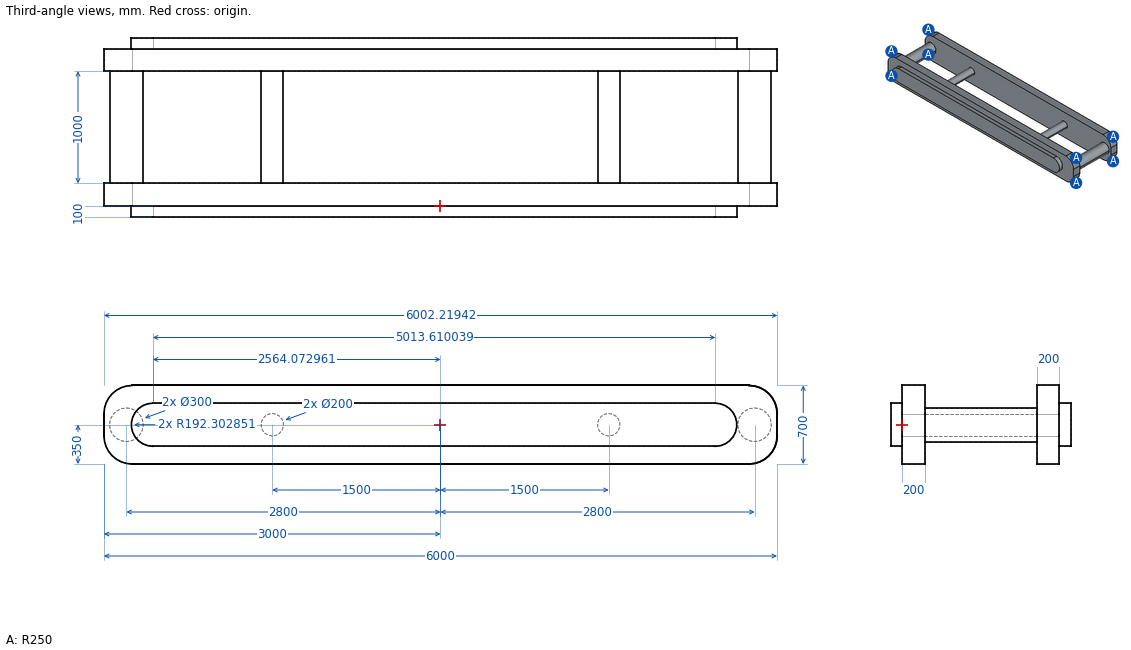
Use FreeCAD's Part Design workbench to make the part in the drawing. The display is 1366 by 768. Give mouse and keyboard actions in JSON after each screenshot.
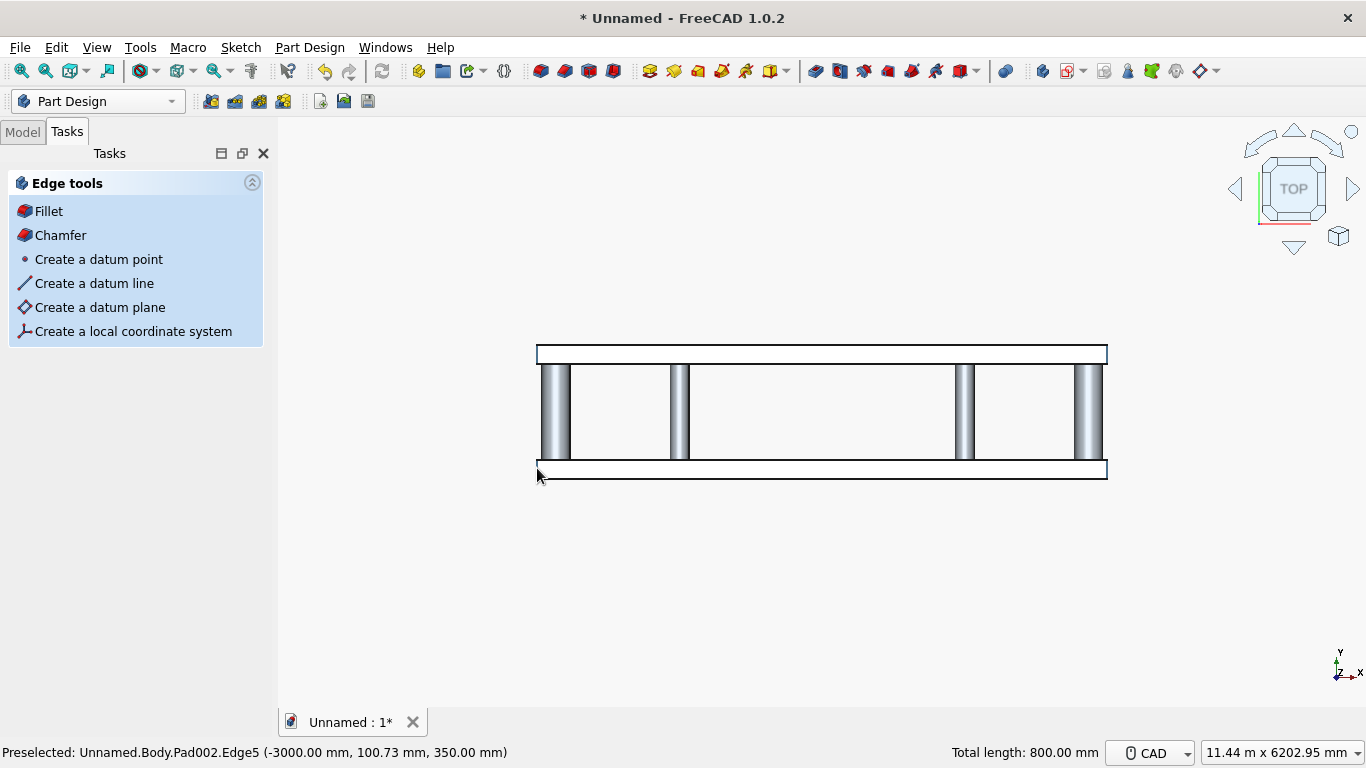
{"action": "scroll", "coordinate": [1107, 354], "scroll_direction": "up", "scroll_amount": 4}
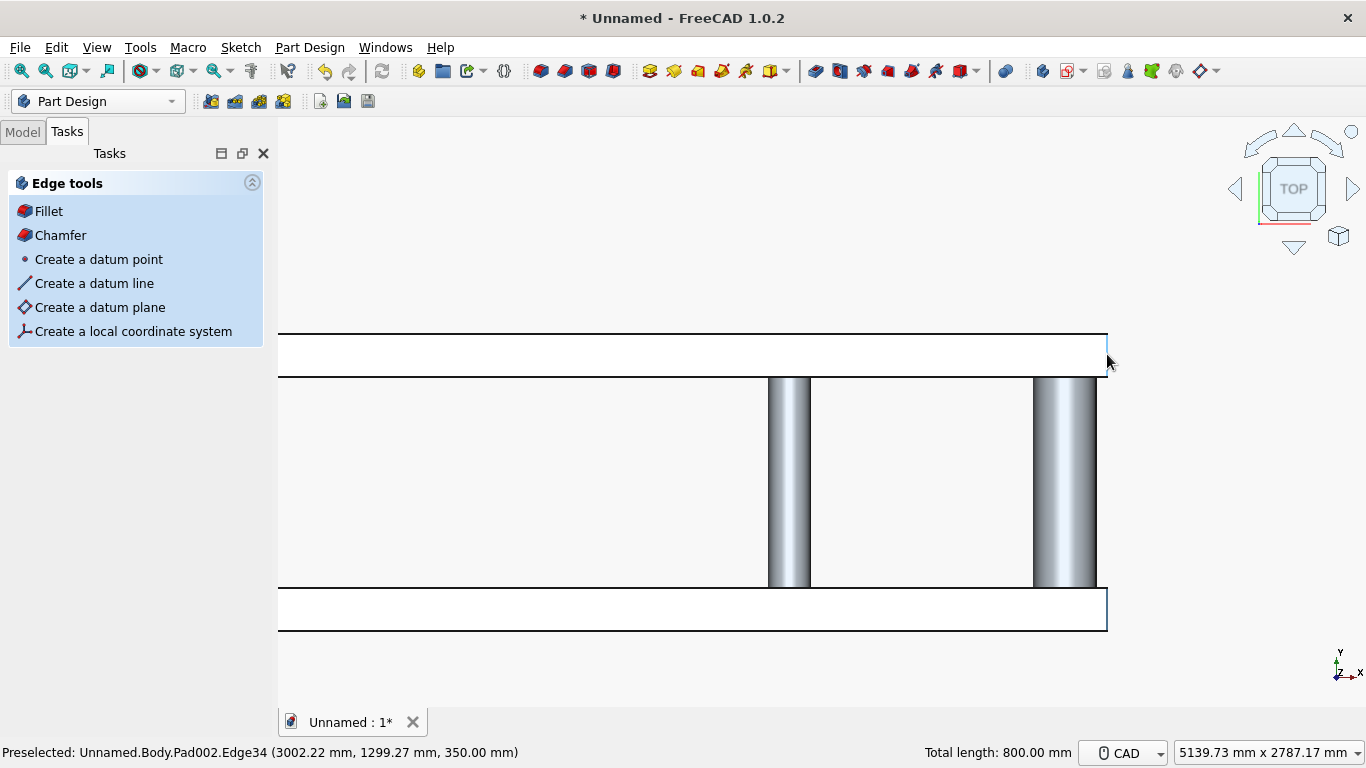
{"action": "left_click", "coordinate": [22, 72]}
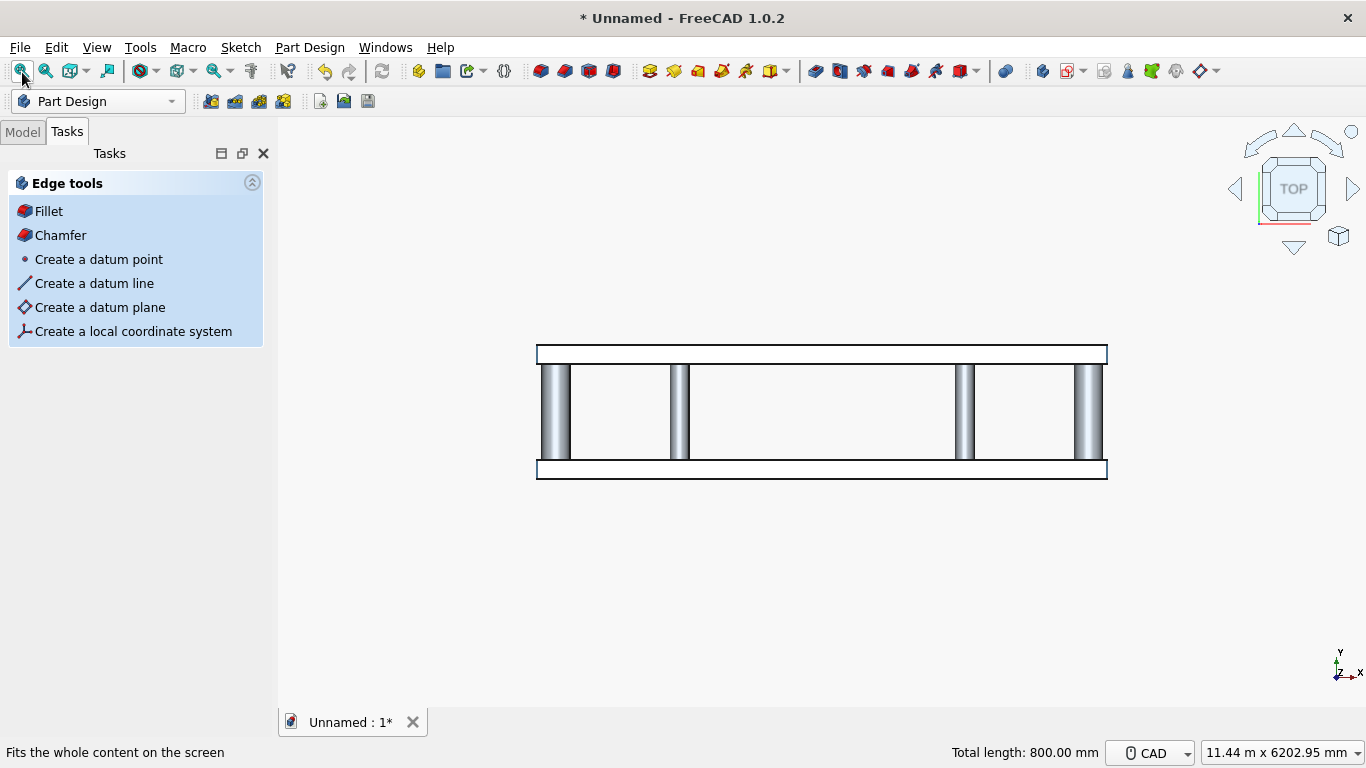
{"action": "key", "text": "1"}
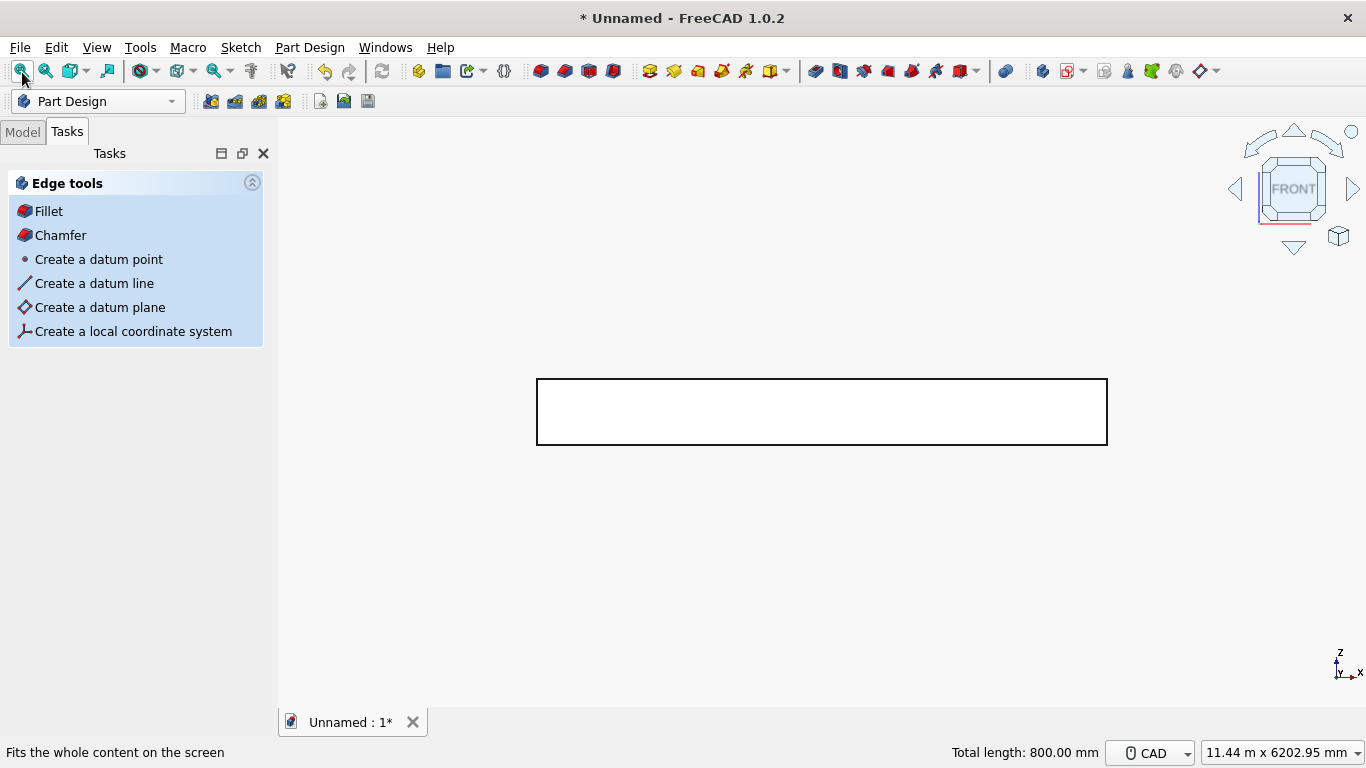
{"action": "scroll", "coordinate": [1107, 444], "scroll_direction": "up", "scroll_amount": 4}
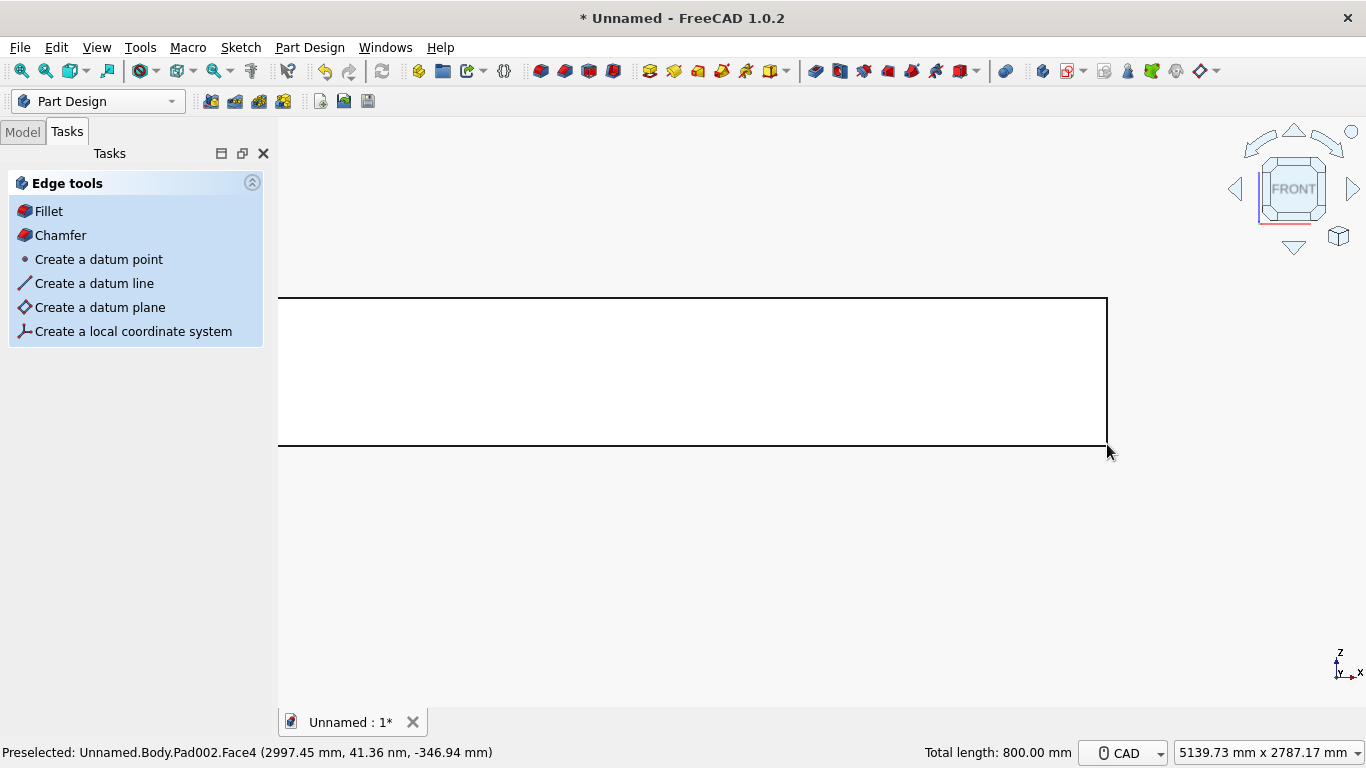
{"action": "left_click", "coordinate": [22, 72]}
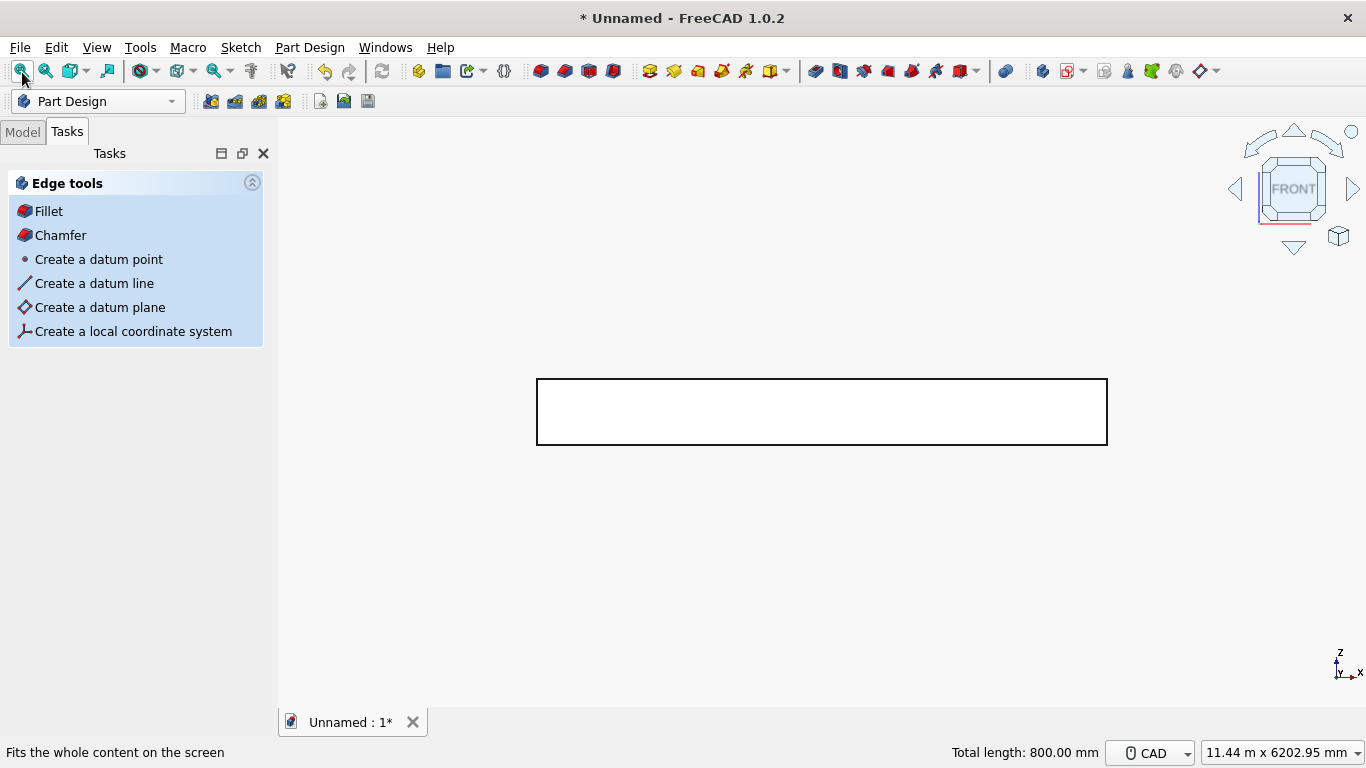
{"action": "key", "text": "3"}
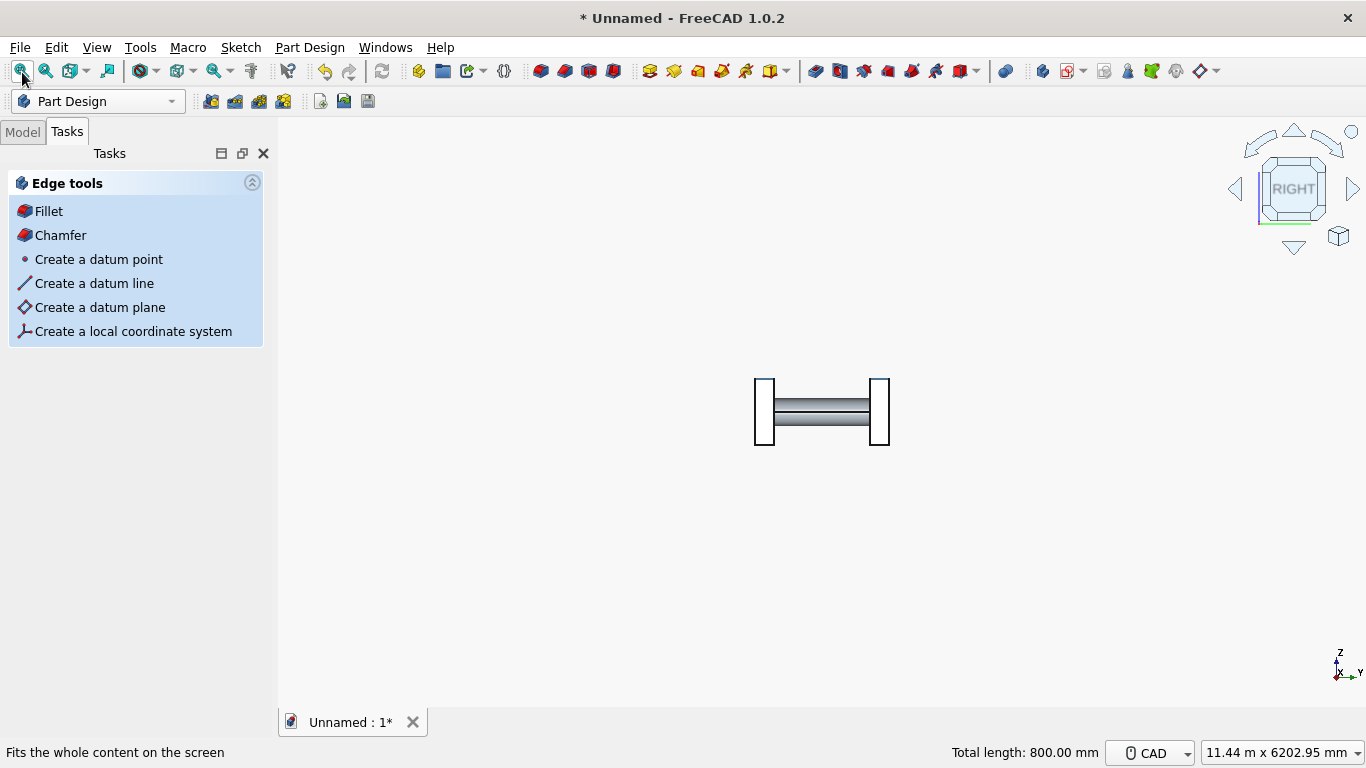
{"action": "key", "text": "v f"}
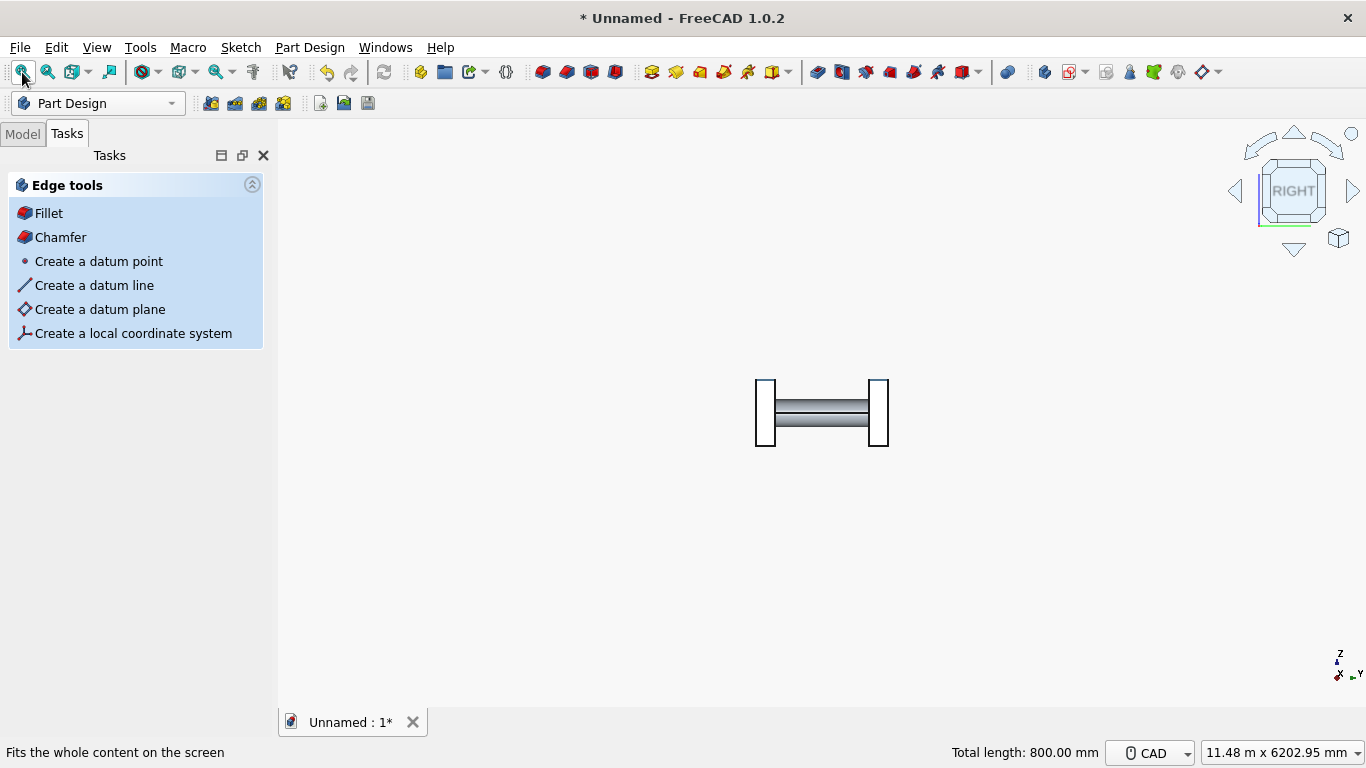
{"action": "left_click", "coordinate": [879, 445], "text": "ctrl"}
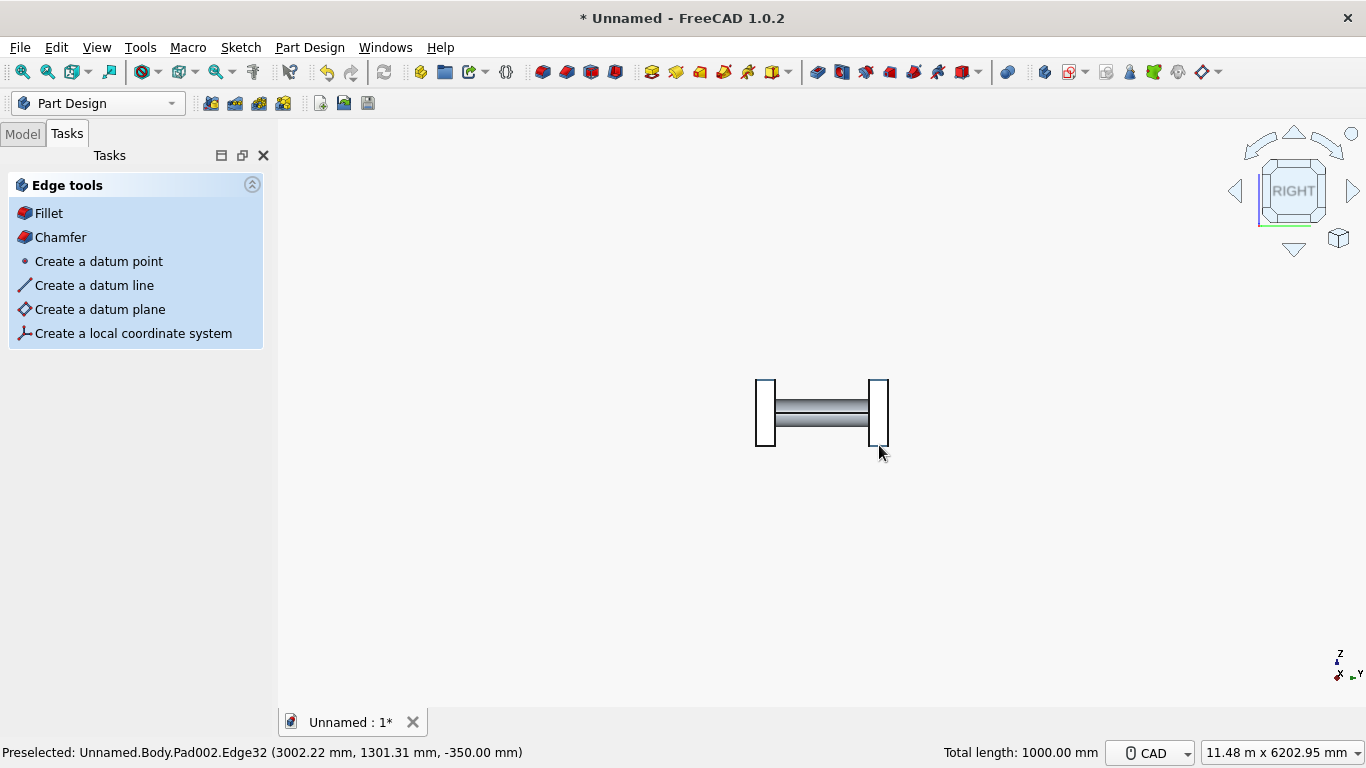
{"action": "left_click", "coordinate": [765, 445], "text": "ctrl"}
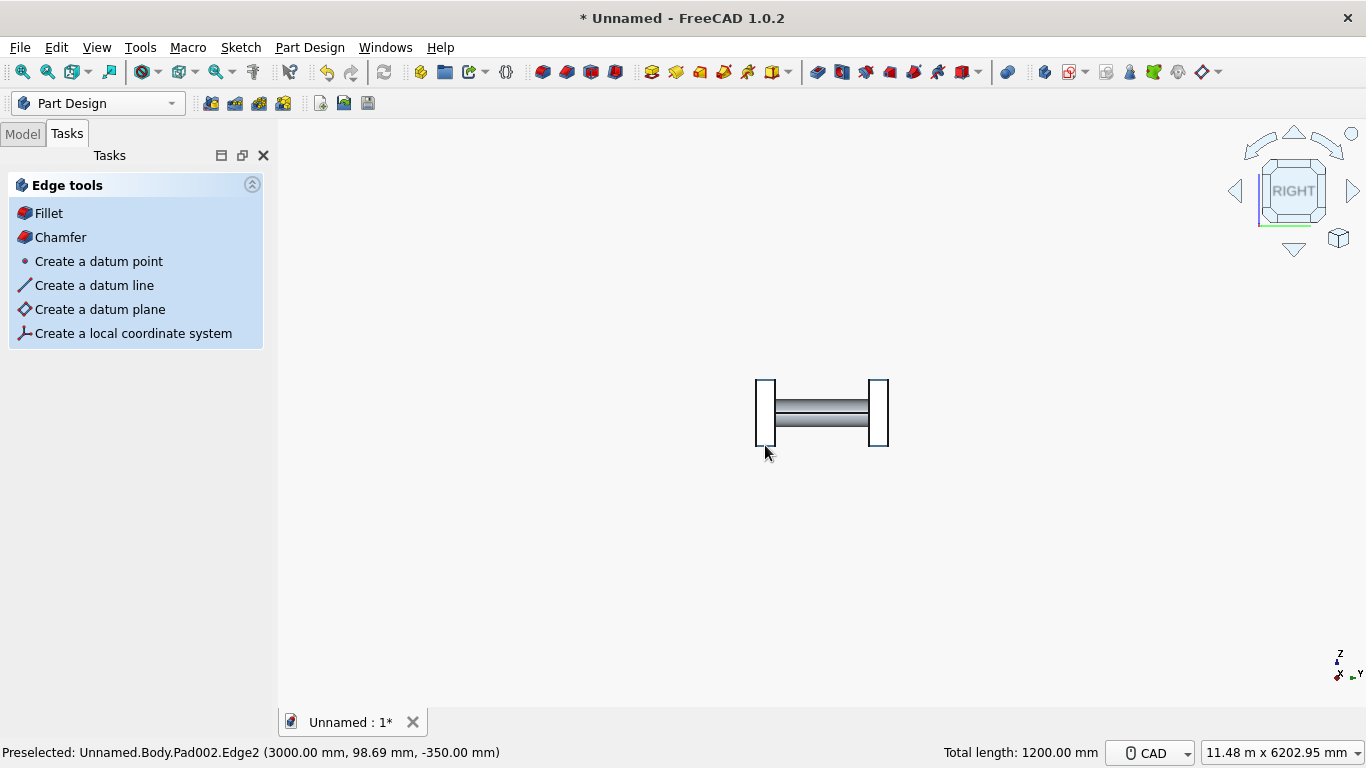
{"action": "scroll", "coordinate": [879, 445], "scroll_direction": "up", "scroll_amount": 4}